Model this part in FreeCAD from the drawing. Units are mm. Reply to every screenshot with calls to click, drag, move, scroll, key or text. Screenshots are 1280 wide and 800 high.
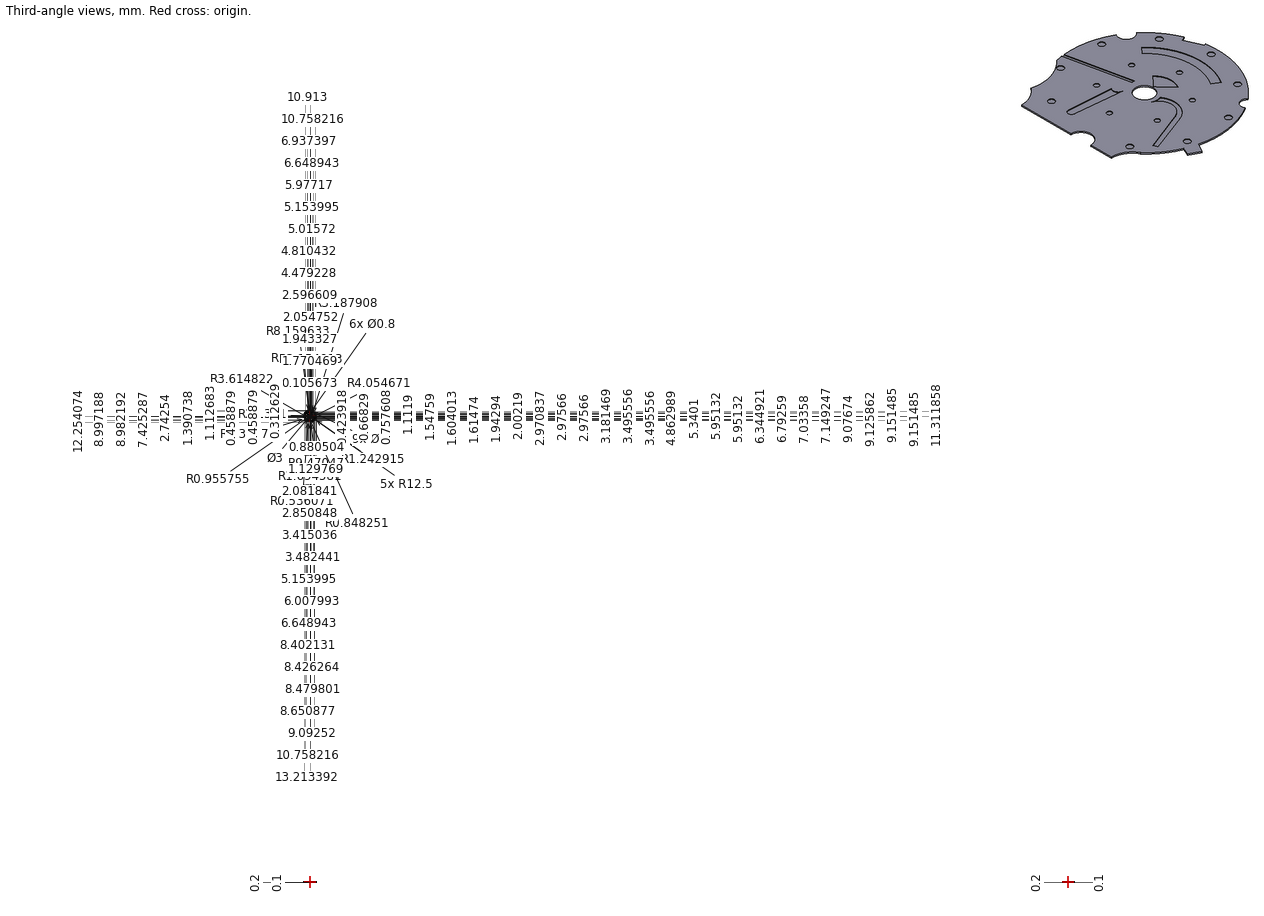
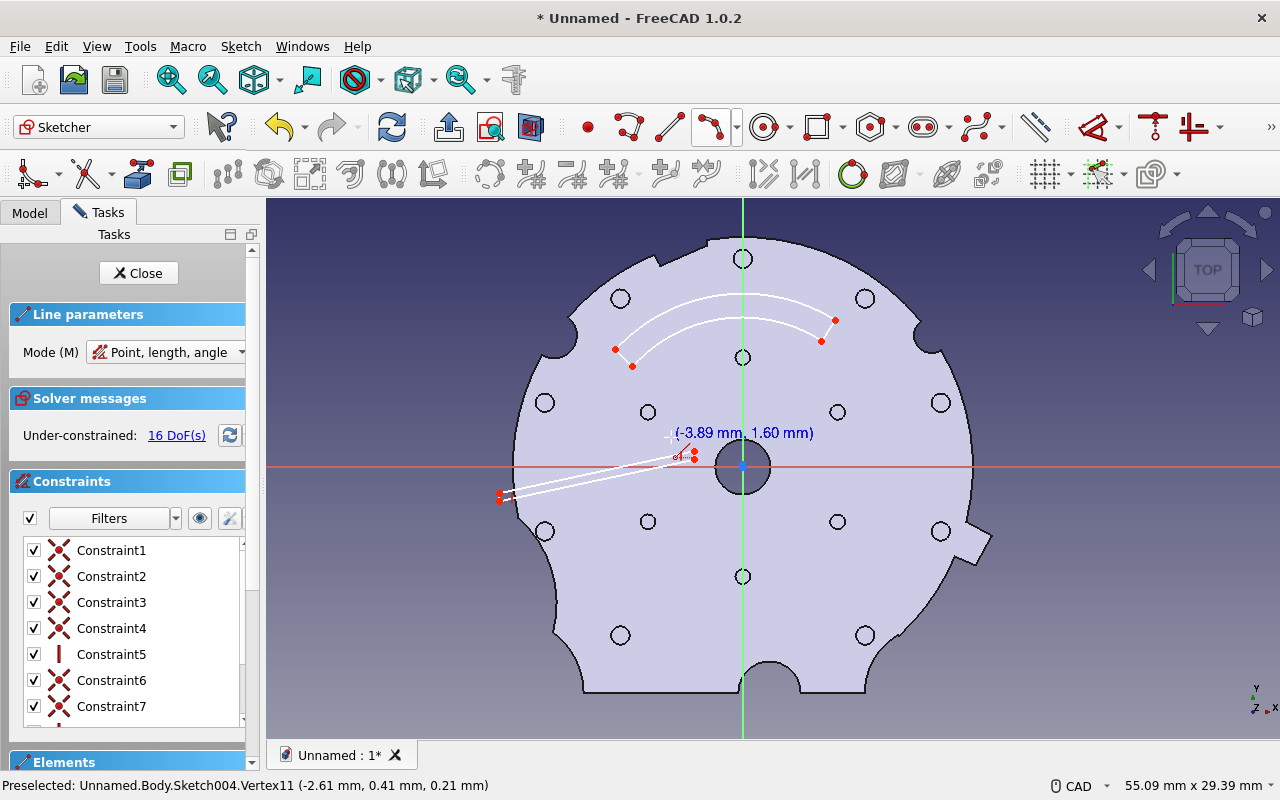
click(690, 634)
click(705, 497)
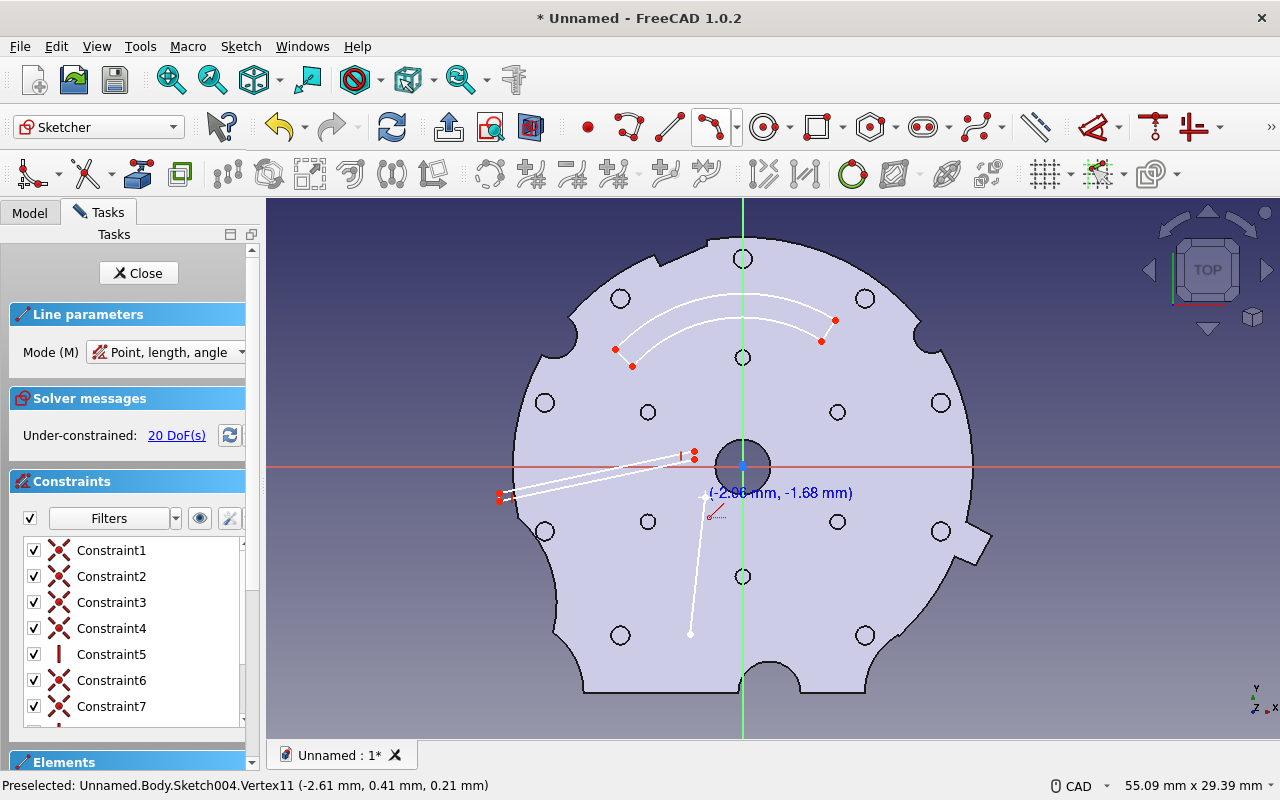
click(680, 508)
click(671, 633)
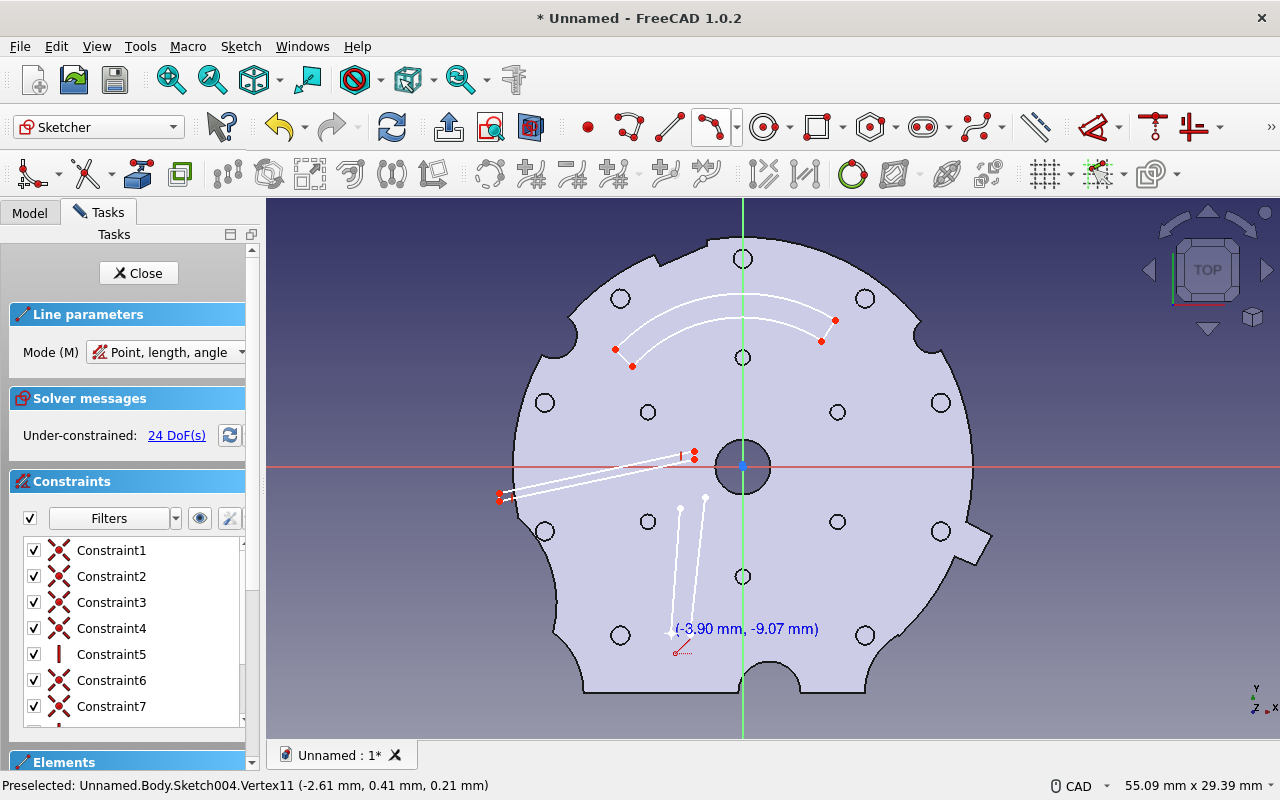
key(g)
key(3)
key(a)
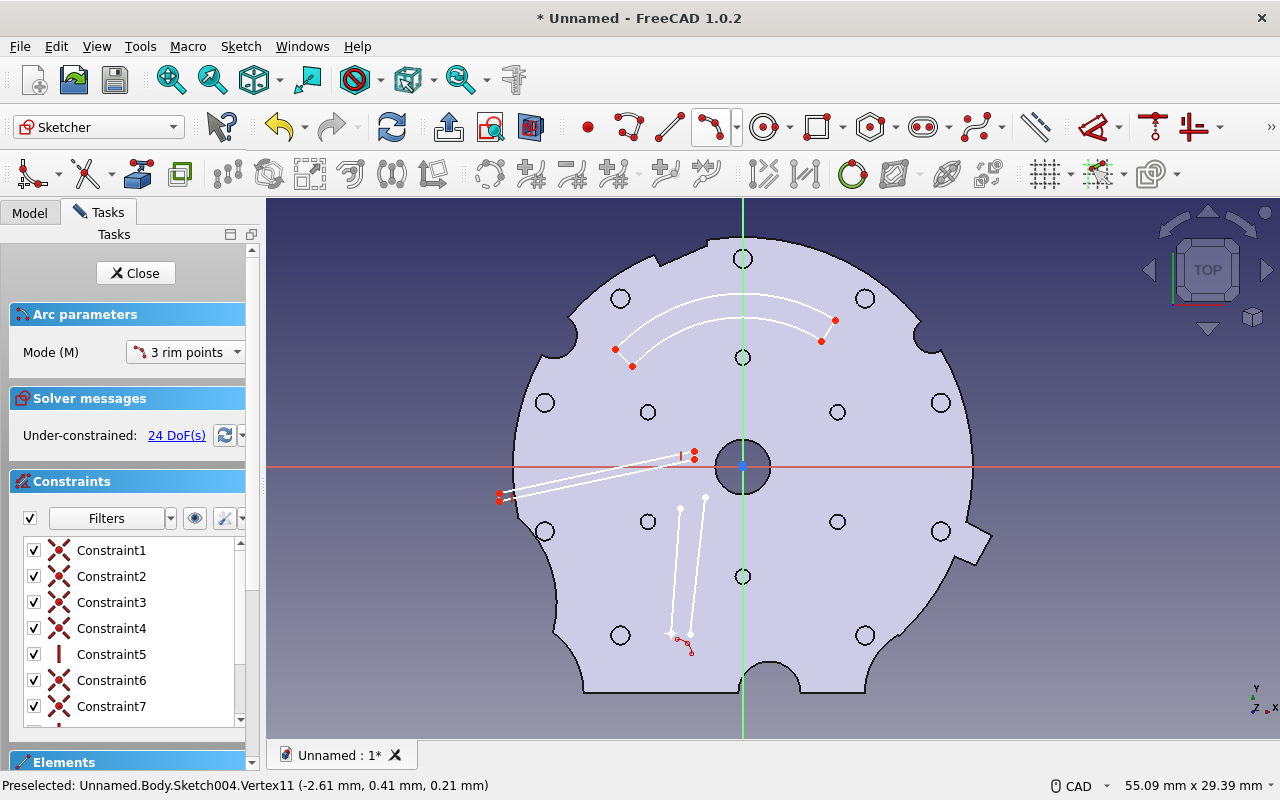
click(705, 498)
click(680, 509)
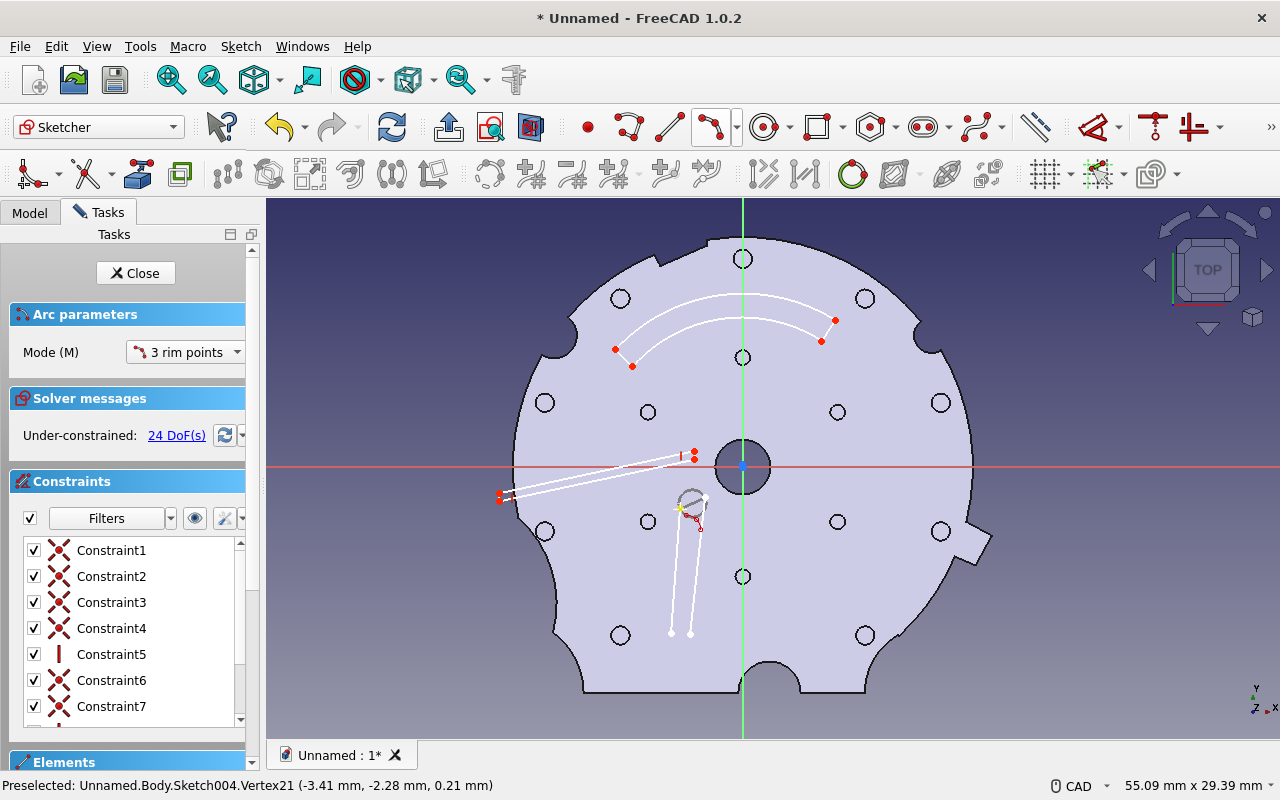
scroll(695, 509, up, 4)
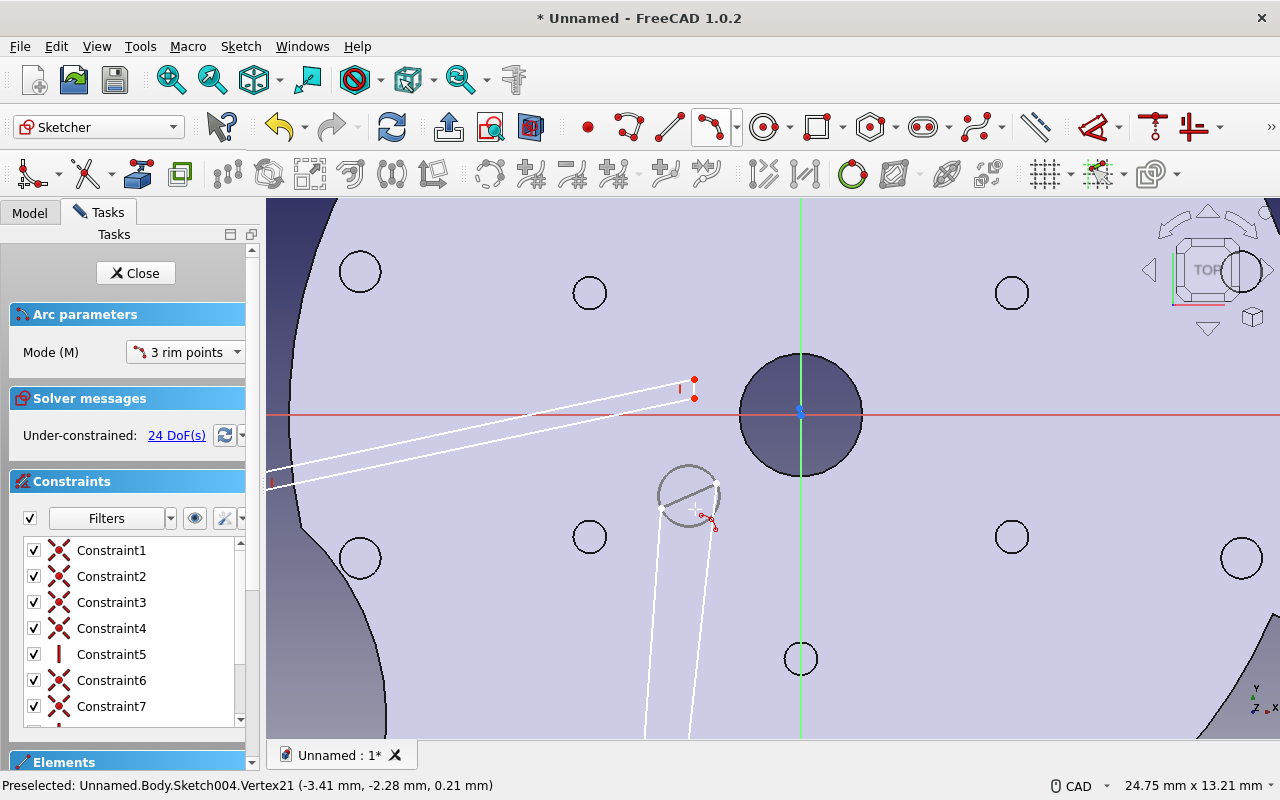
click(695, 509)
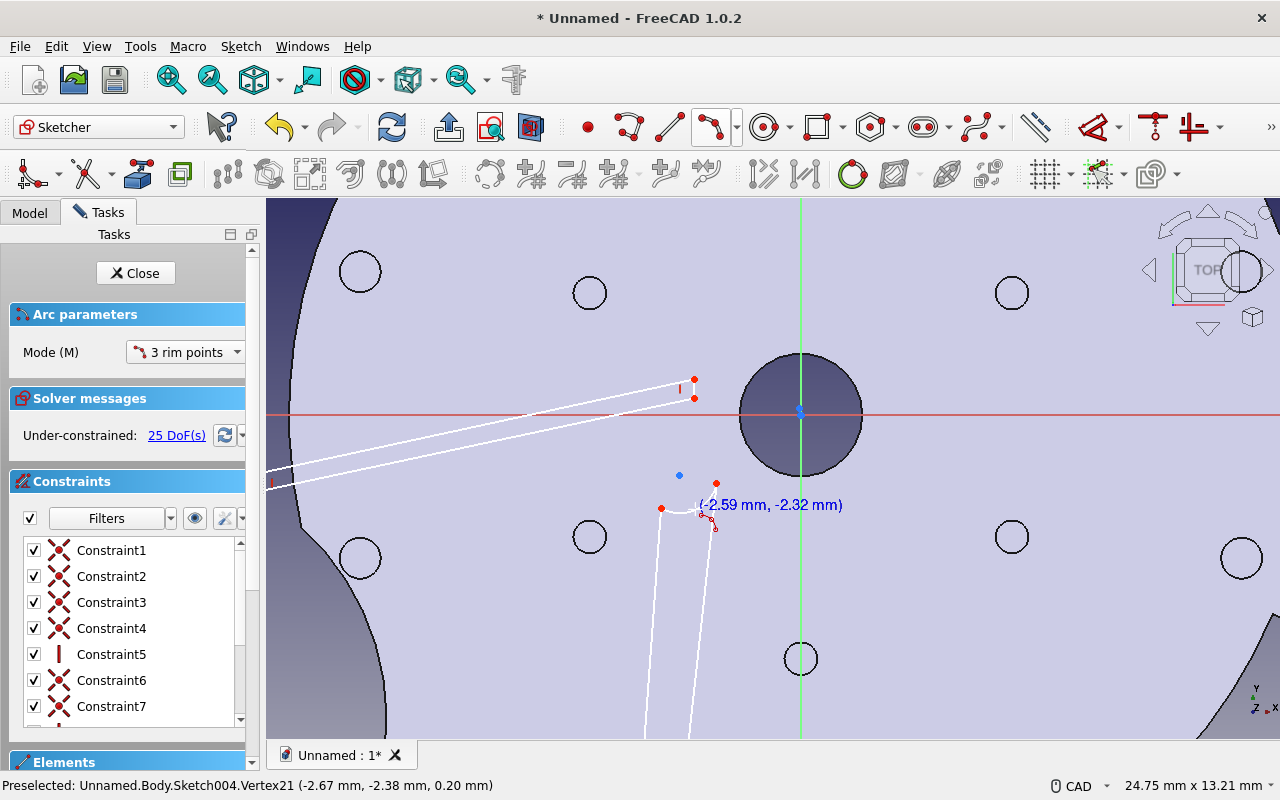
scroll(695, 509, down, 4)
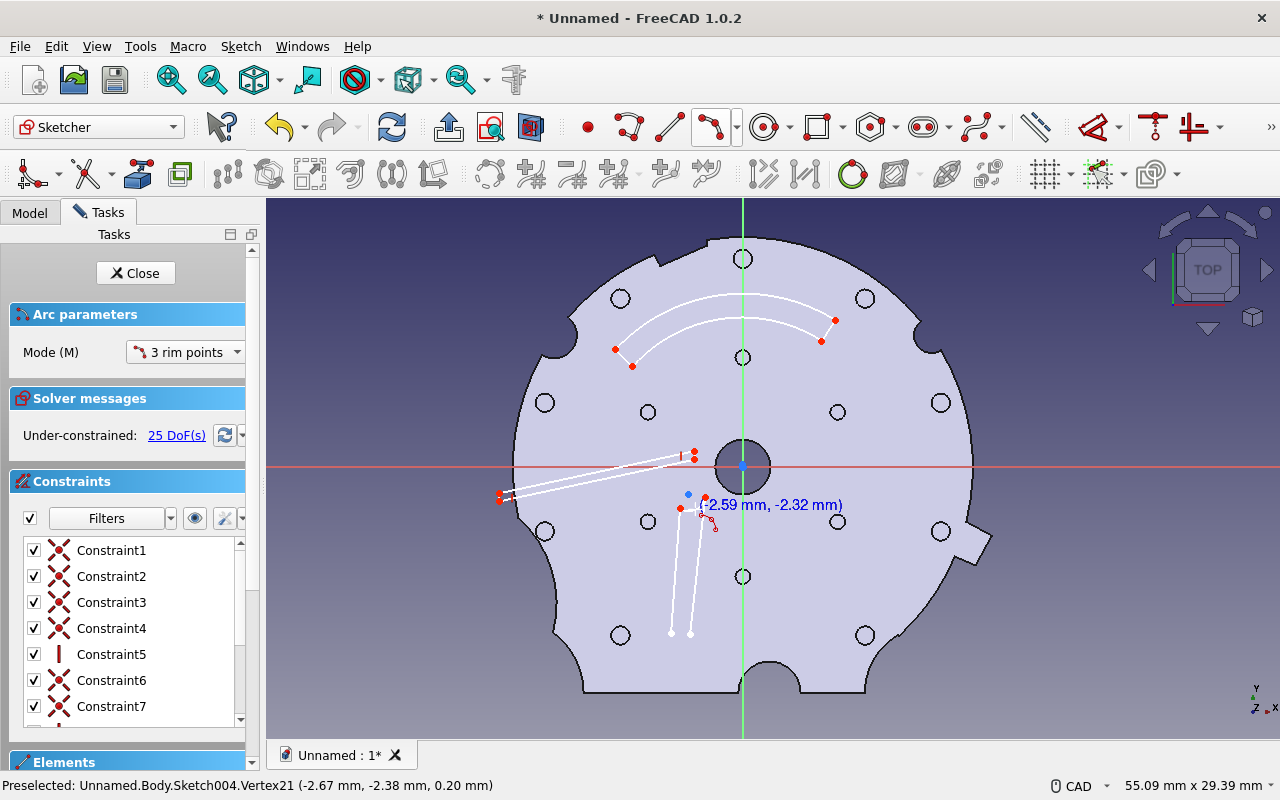
click(671, 634)
click(690, 635)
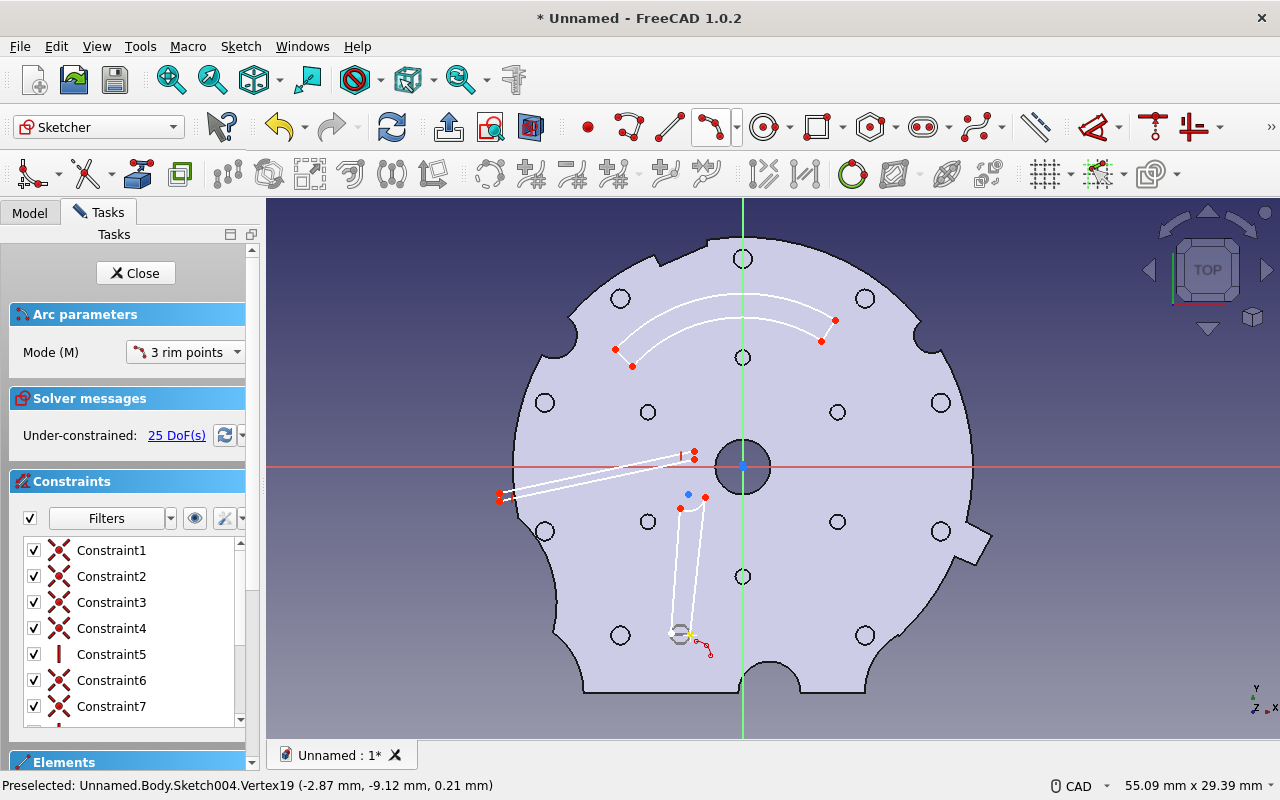
scroll(680, 643, up, 3)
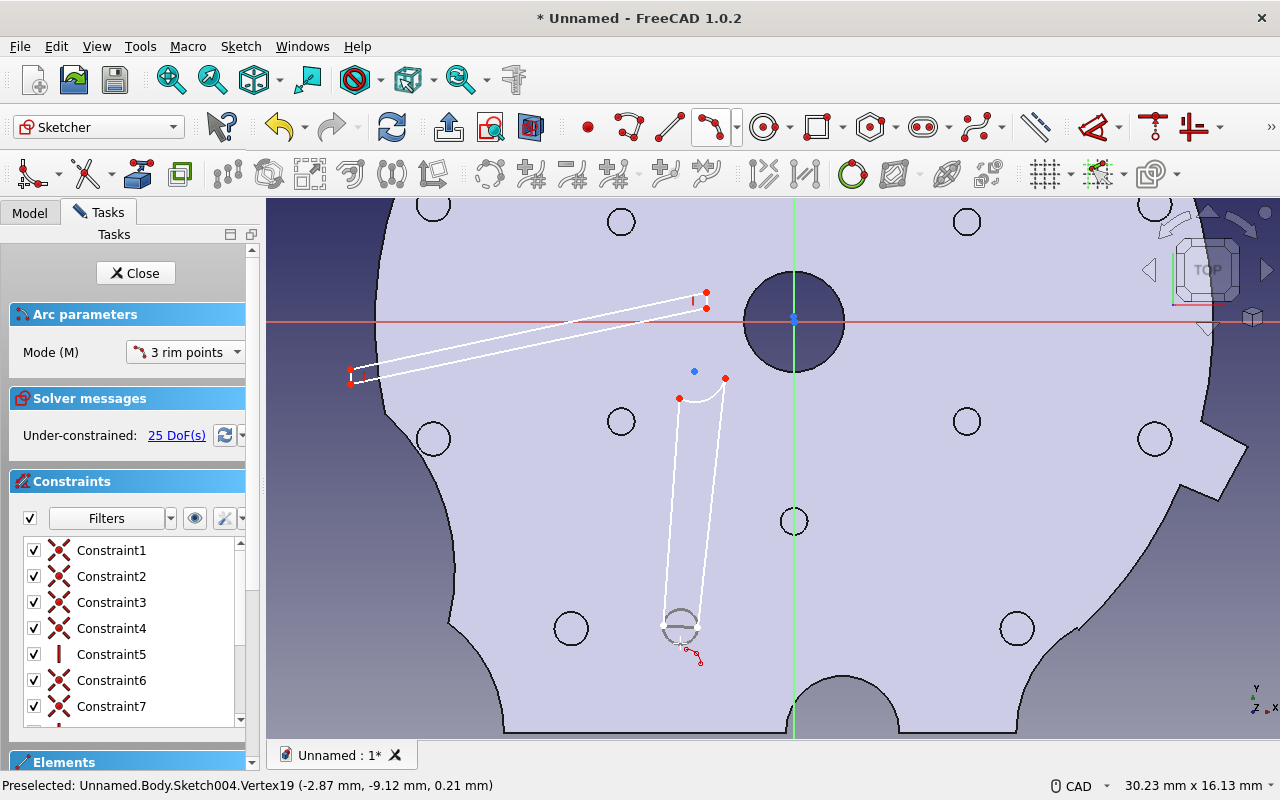
click(679, 643)